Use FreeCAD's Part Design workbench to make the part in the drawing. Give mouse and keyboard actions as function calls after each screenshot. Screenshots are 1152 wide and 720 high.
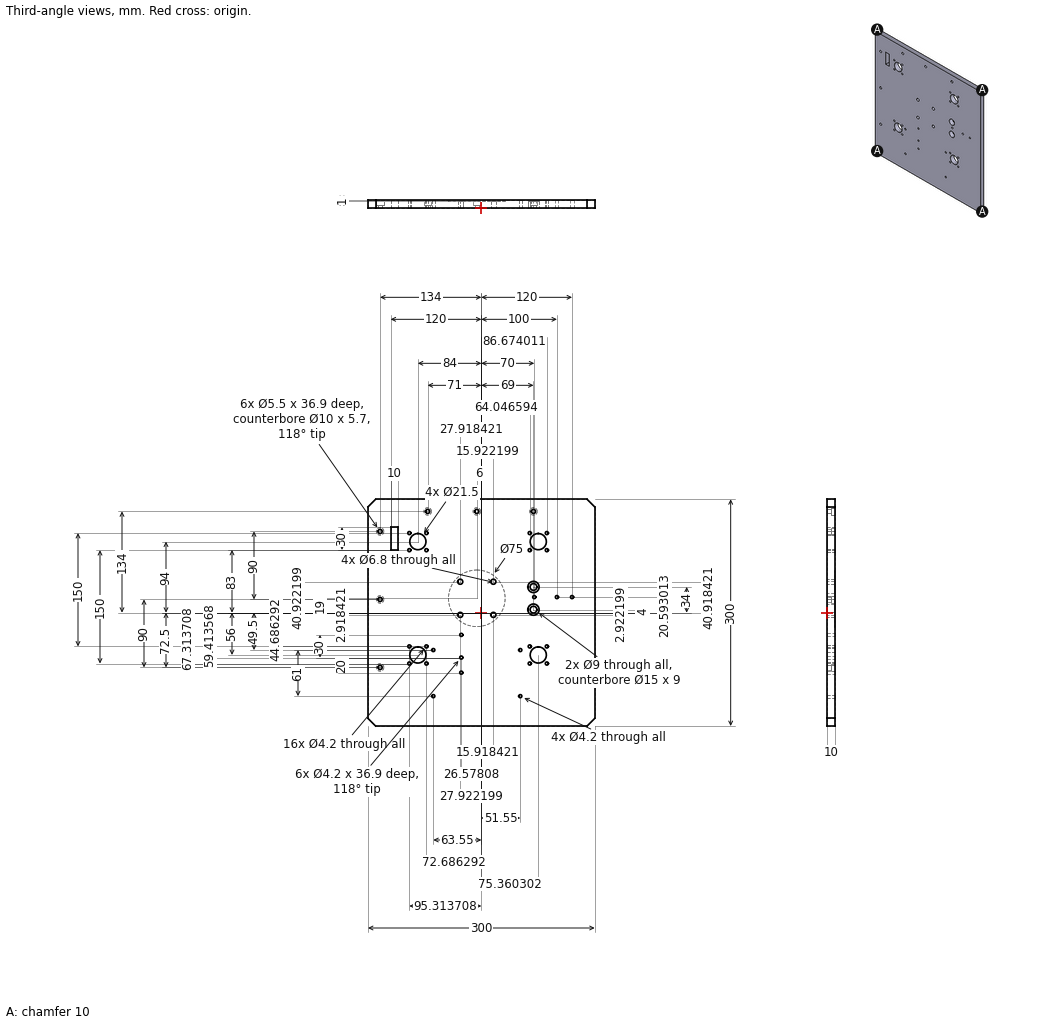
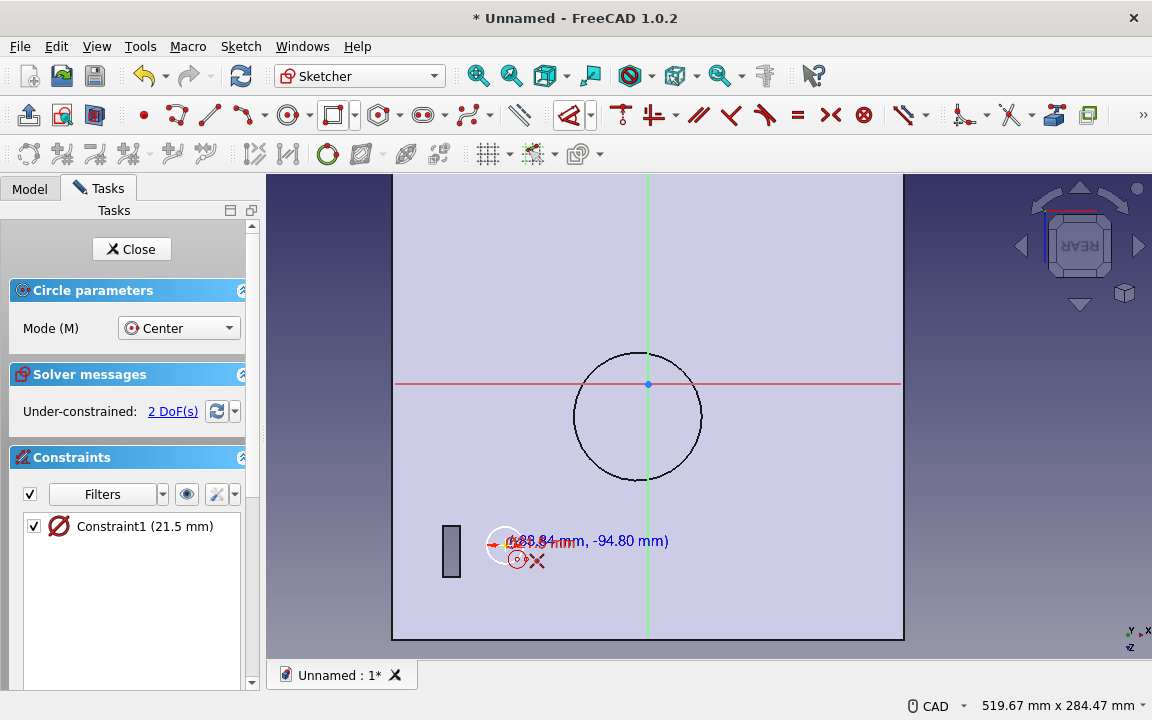
scroll(505, 289, up, 2)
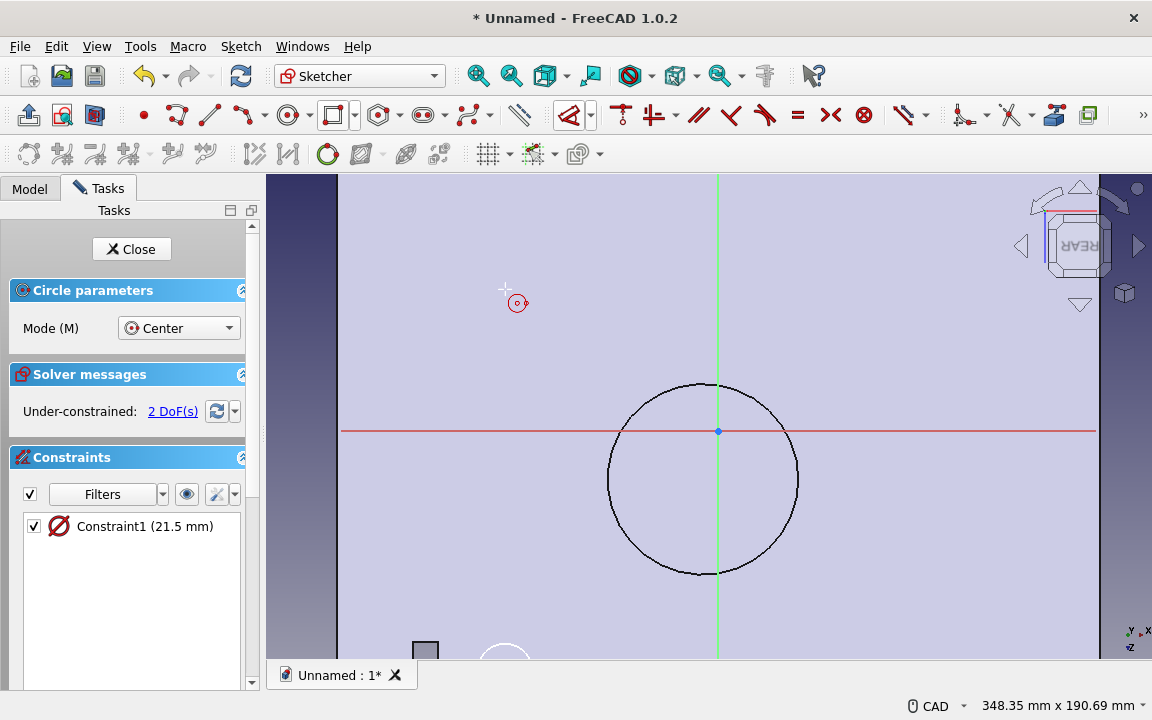
click(505, 289)
move(524, 269)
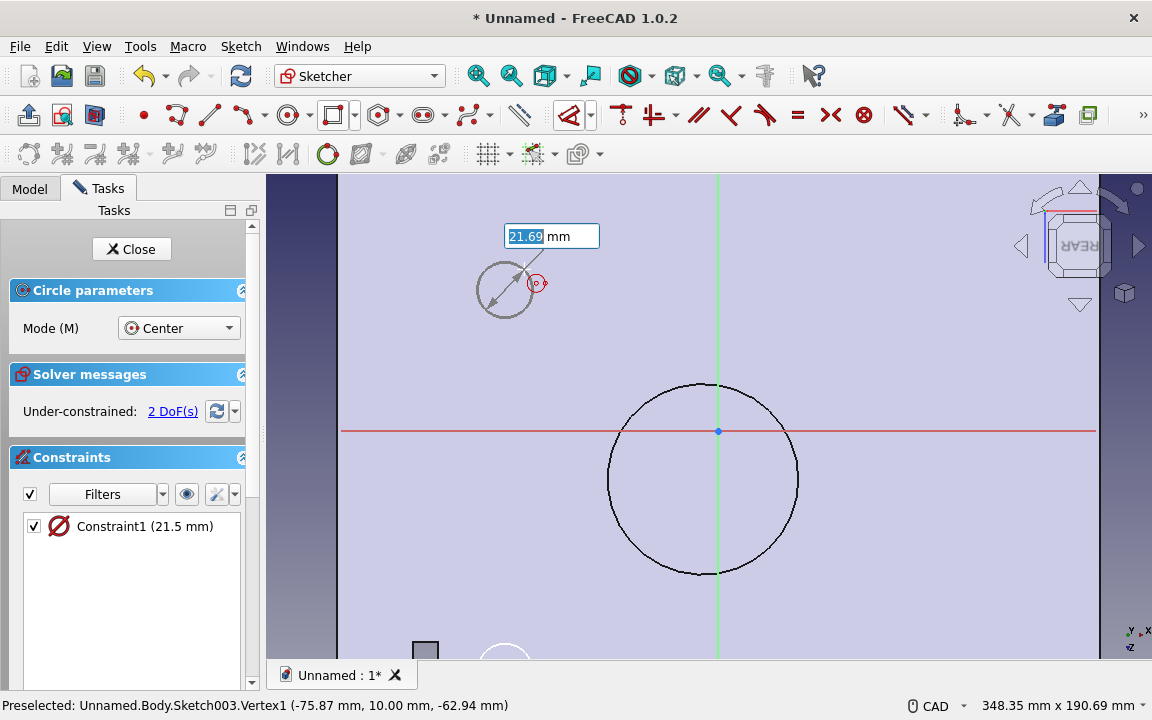
text(21.5)
key(Return)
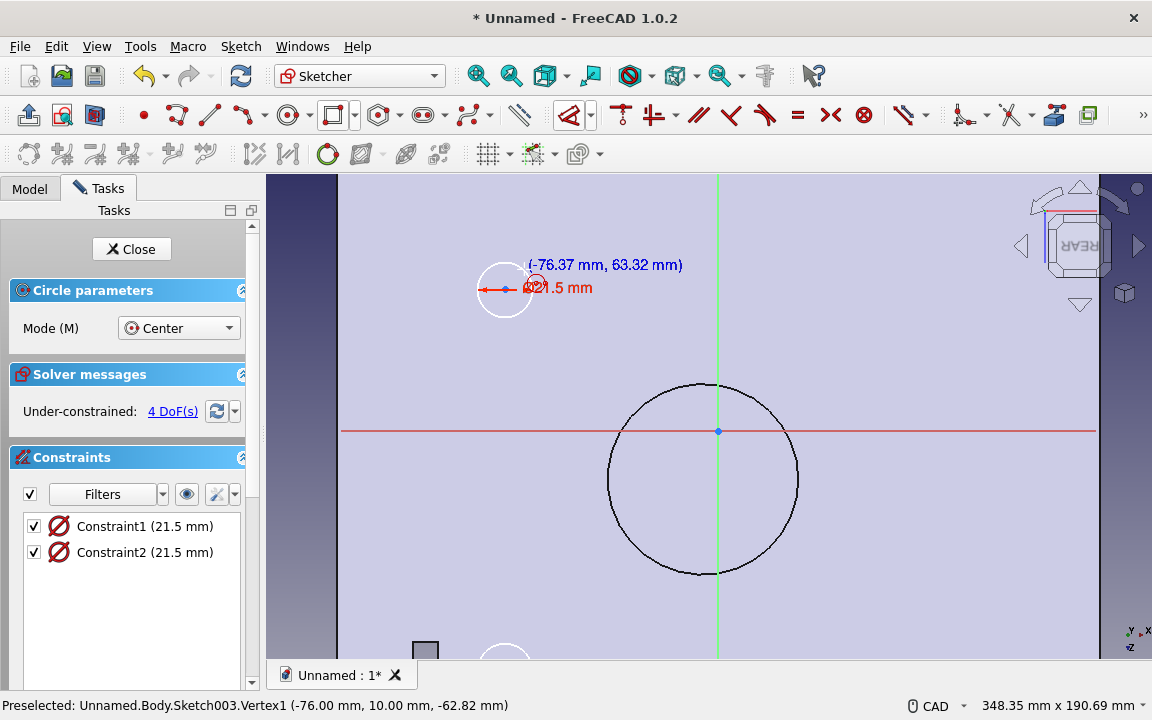
click(910, 289)
move(929, 269)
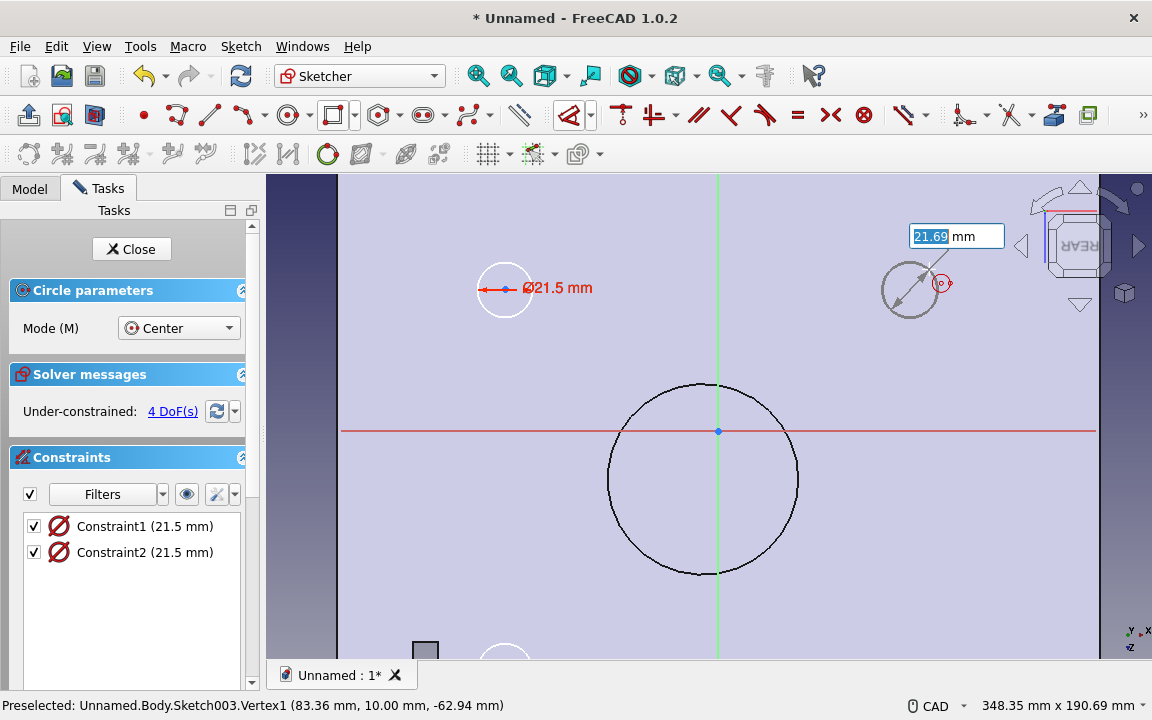
text(21.5)
key(Return)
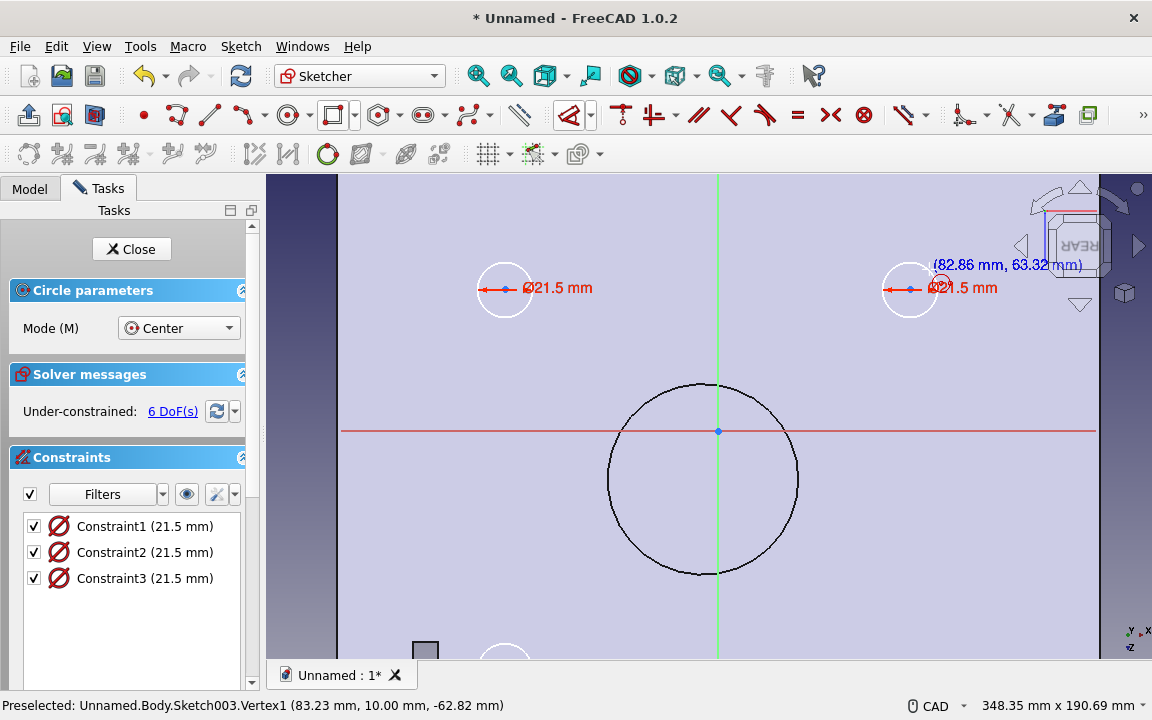
scroll(505, 289, down, 2)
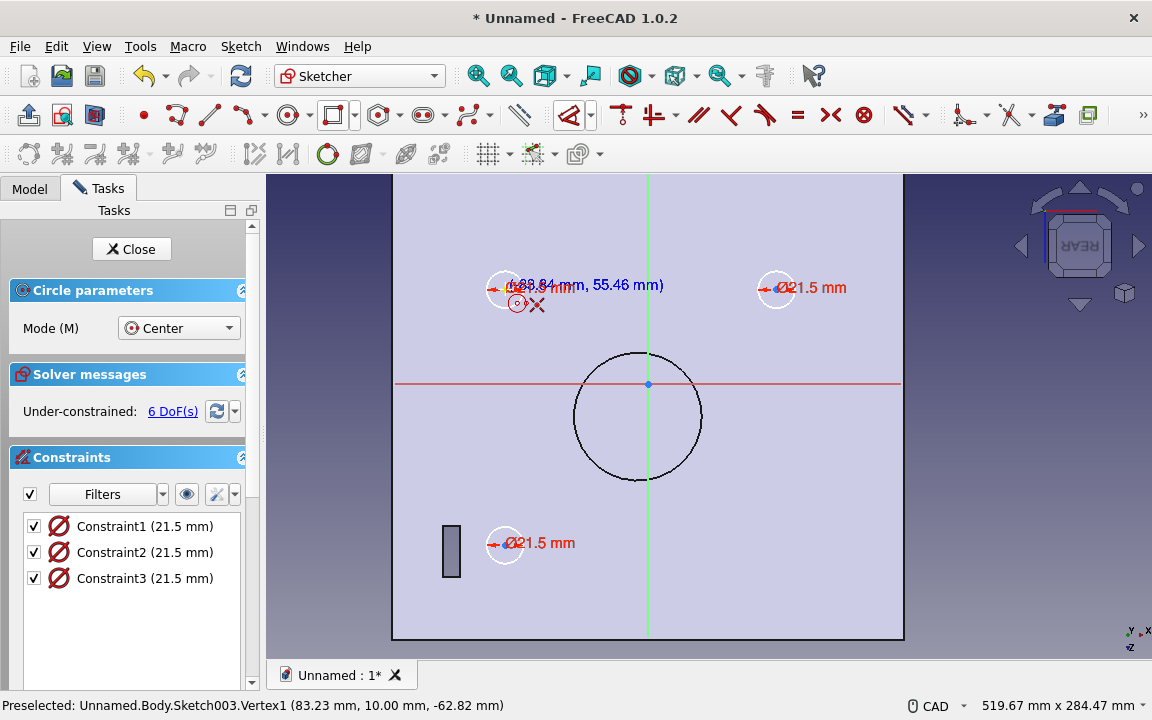
scroll(777, 545, up, 2)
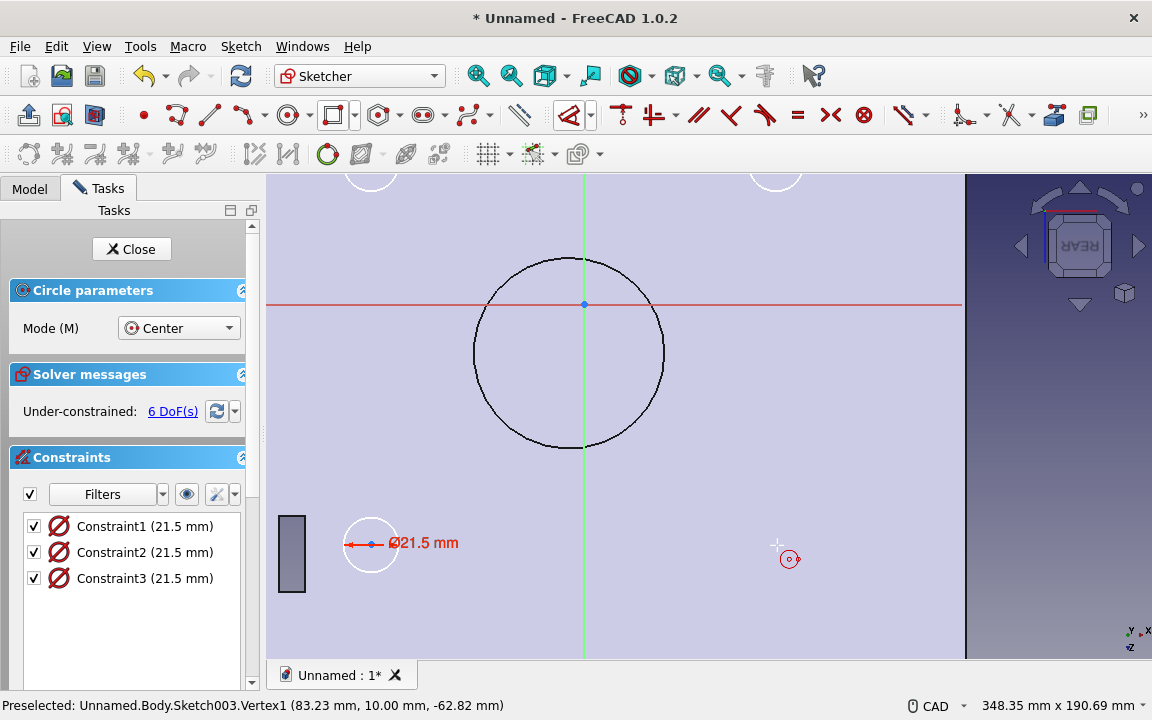
click(776, 544)
move(795, 525)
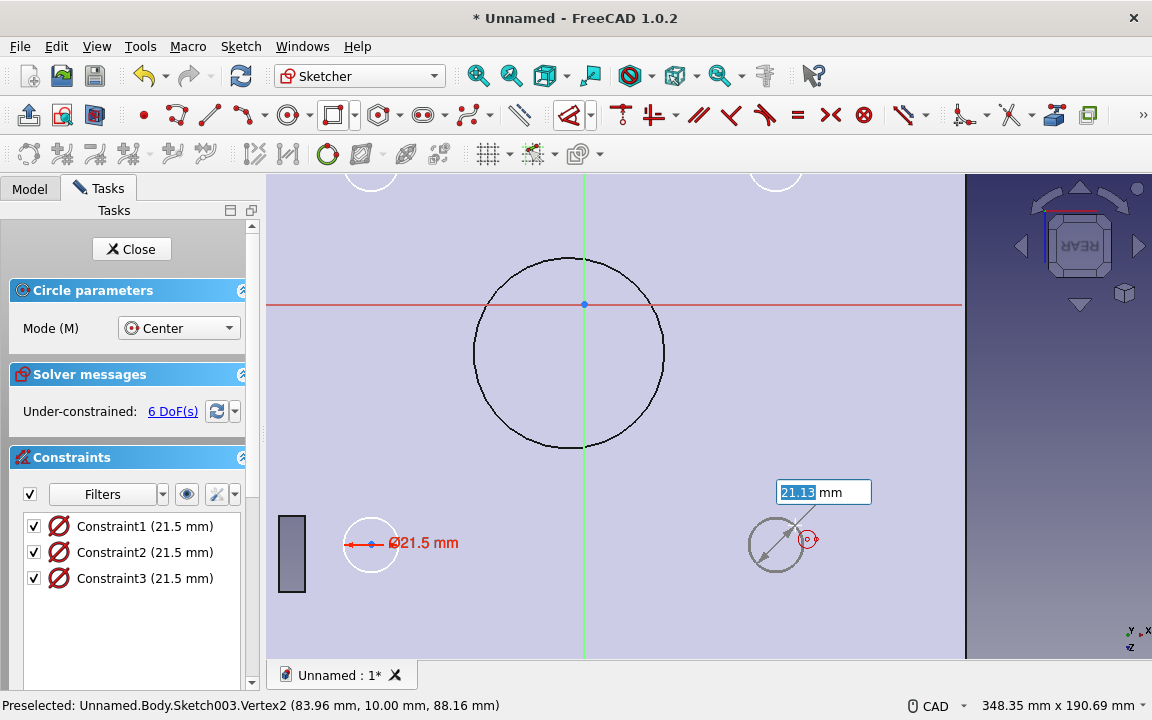
text(21.5)
key(Return)
key(Escape)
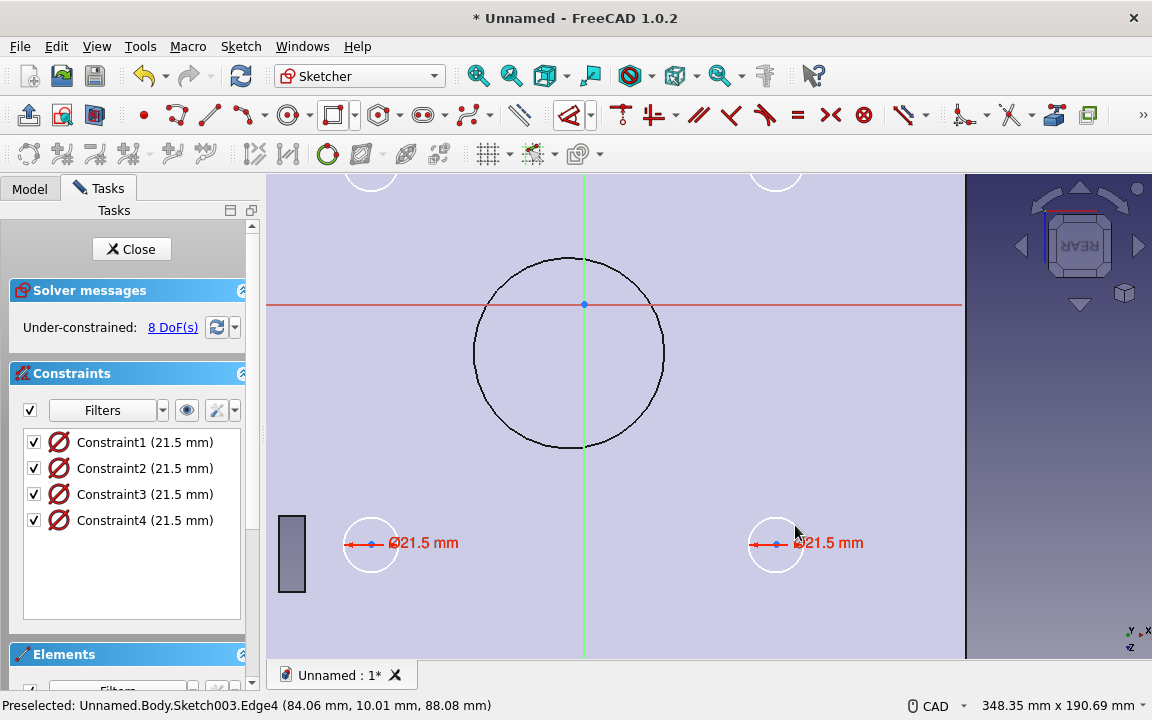
click(371, 545)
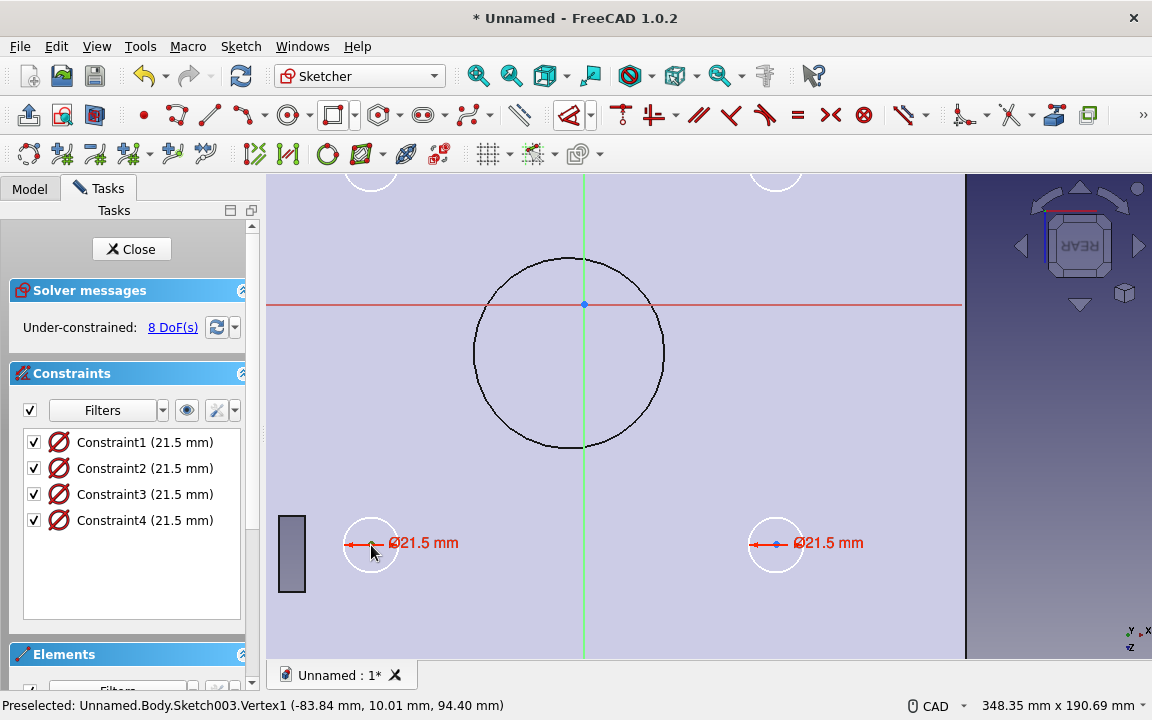
scroll(777, 545, down, 2)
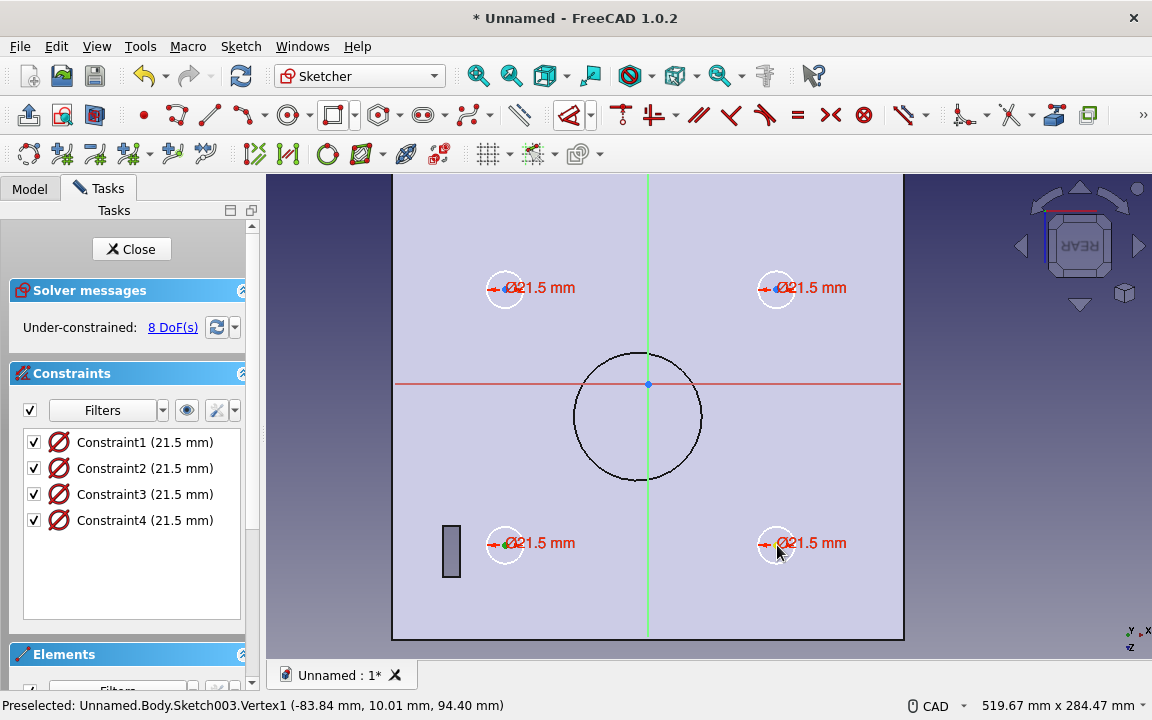
click(505, 290)